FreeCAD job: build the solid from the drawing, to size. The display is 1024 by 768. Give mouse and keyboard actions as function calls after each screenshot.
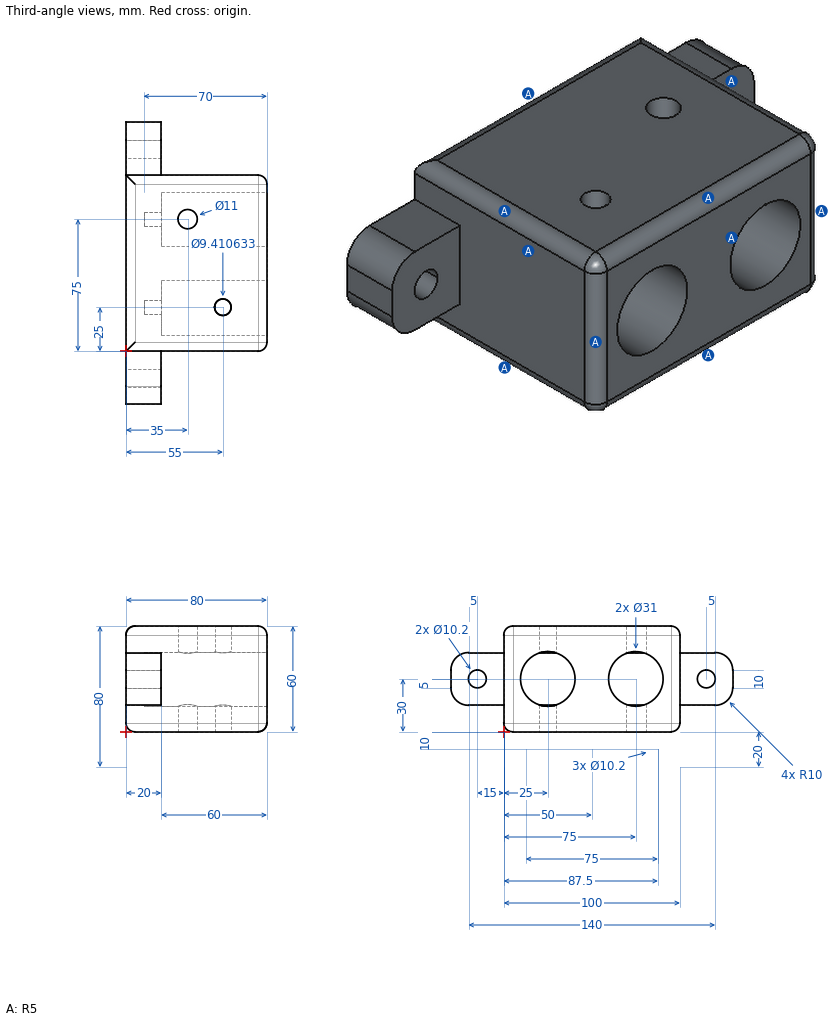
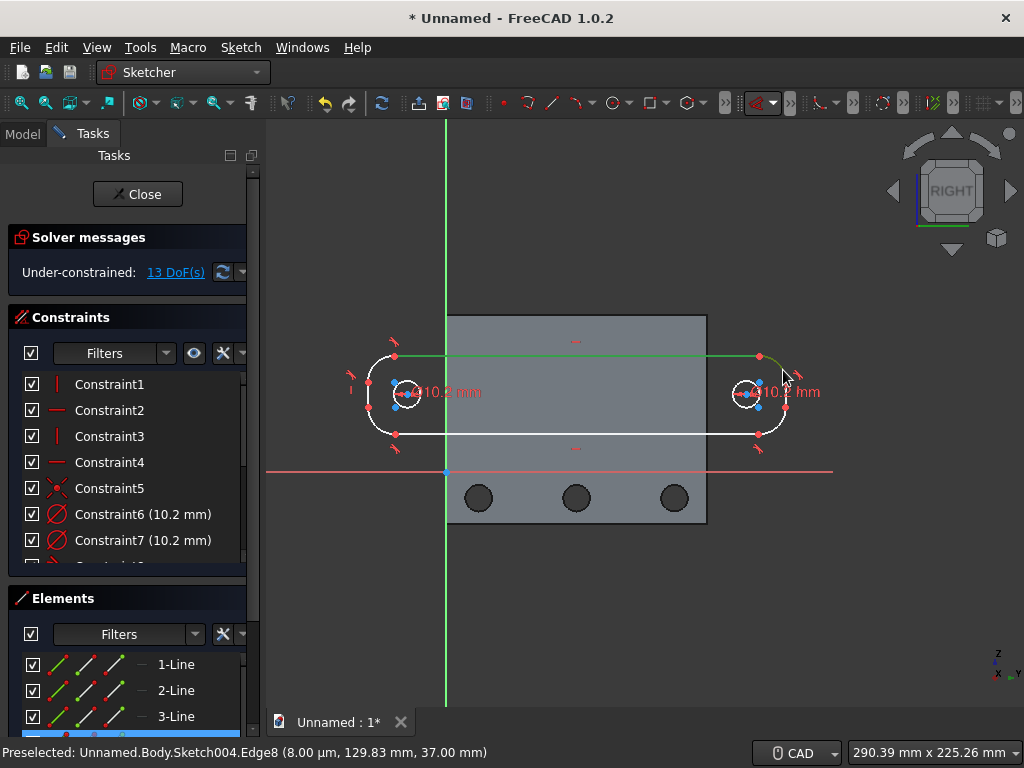
key(t)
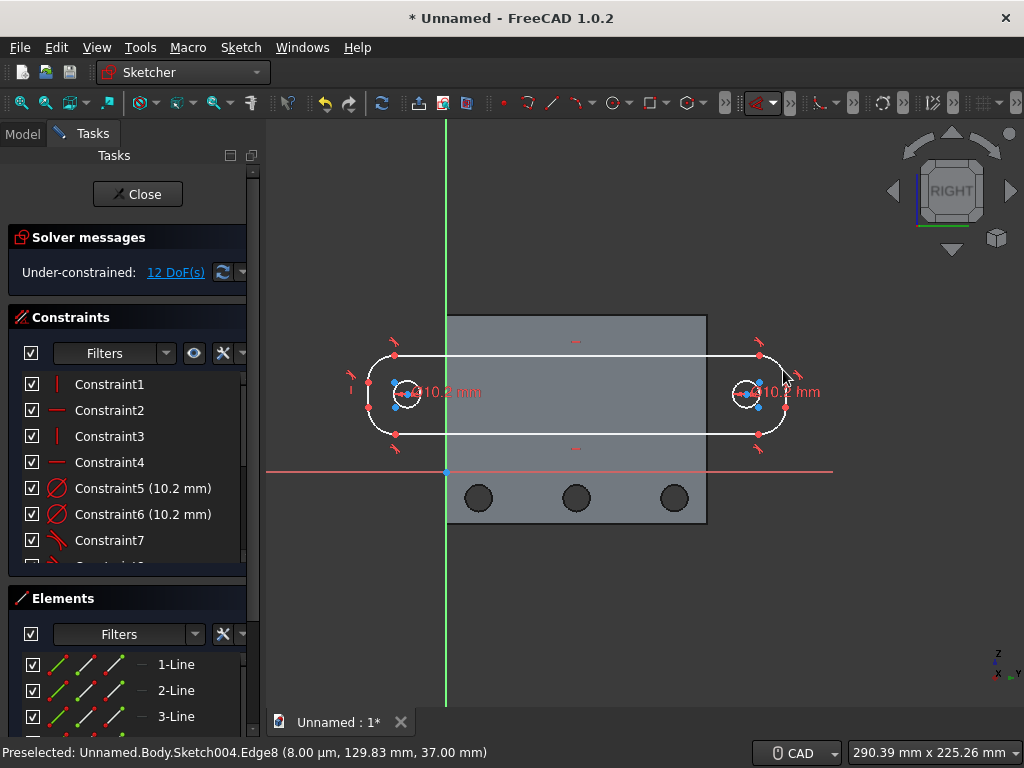
click(771, 431)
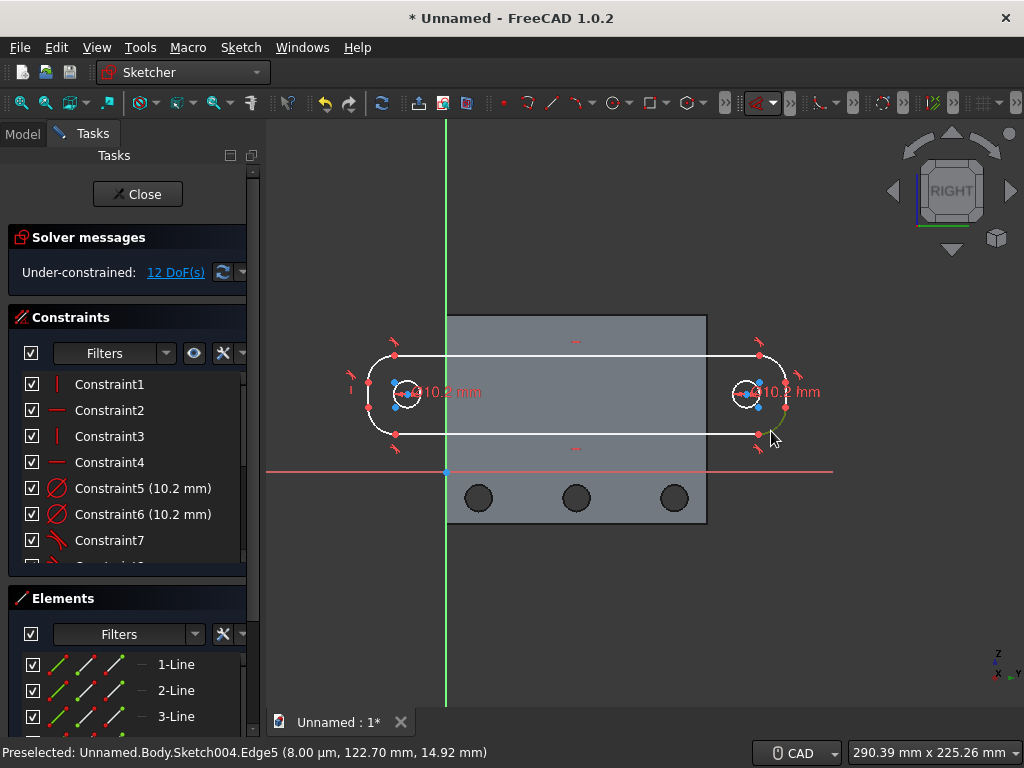
click(371, 419)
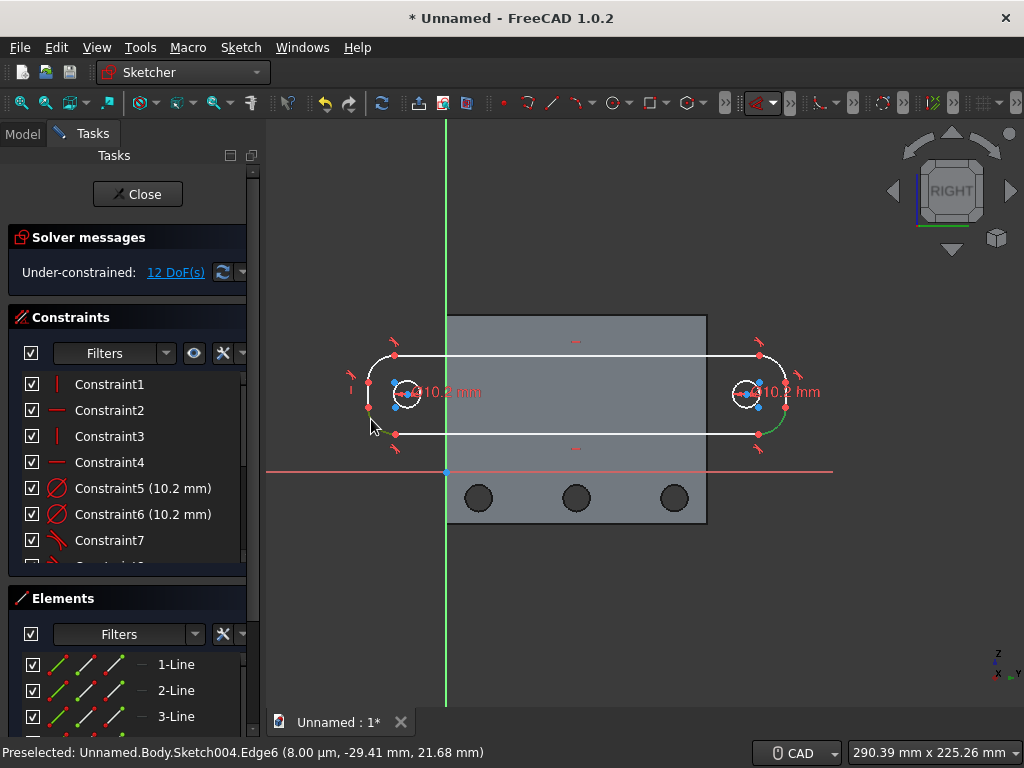
click(382, 359)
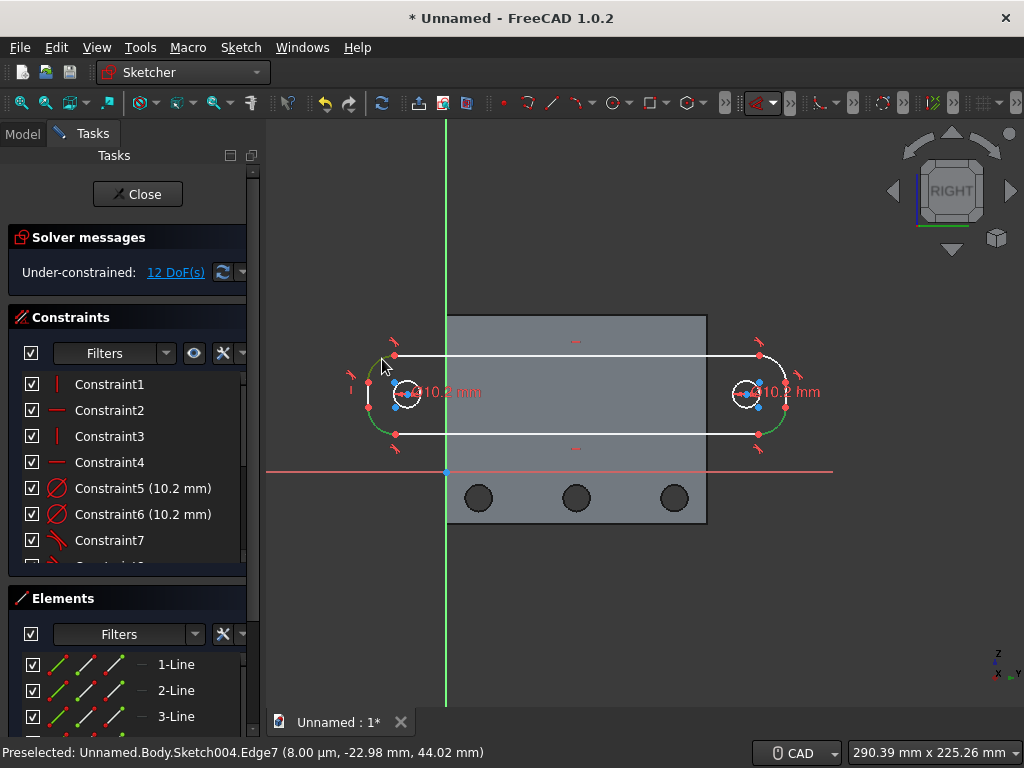
click(783, 370)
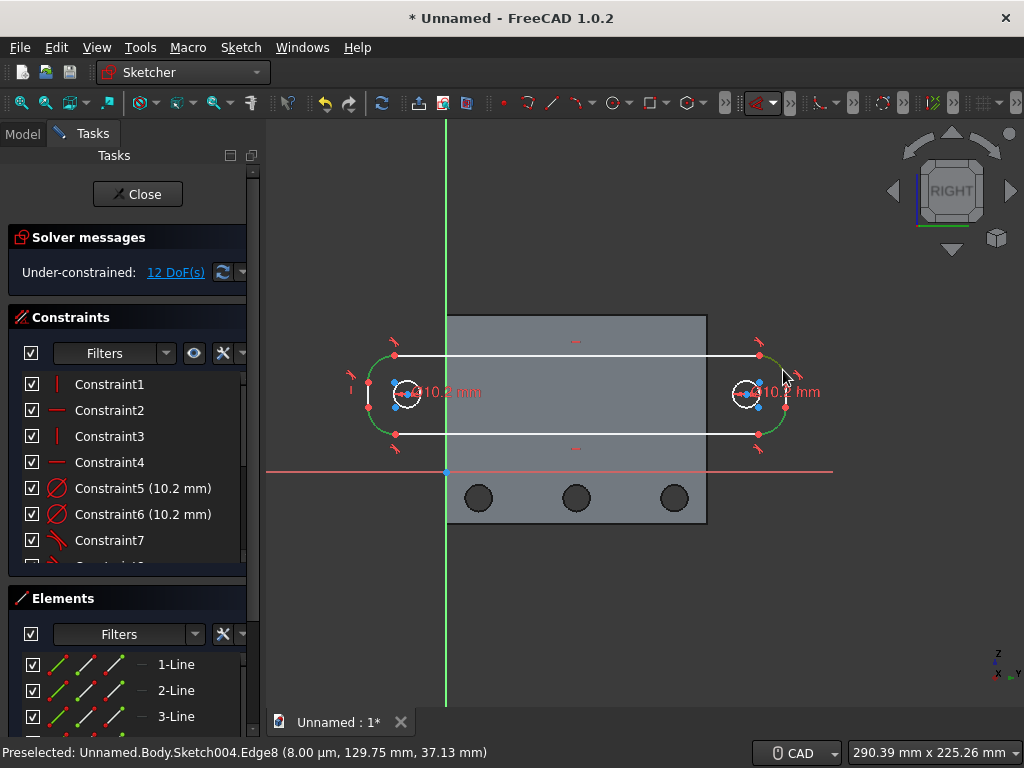
key(e)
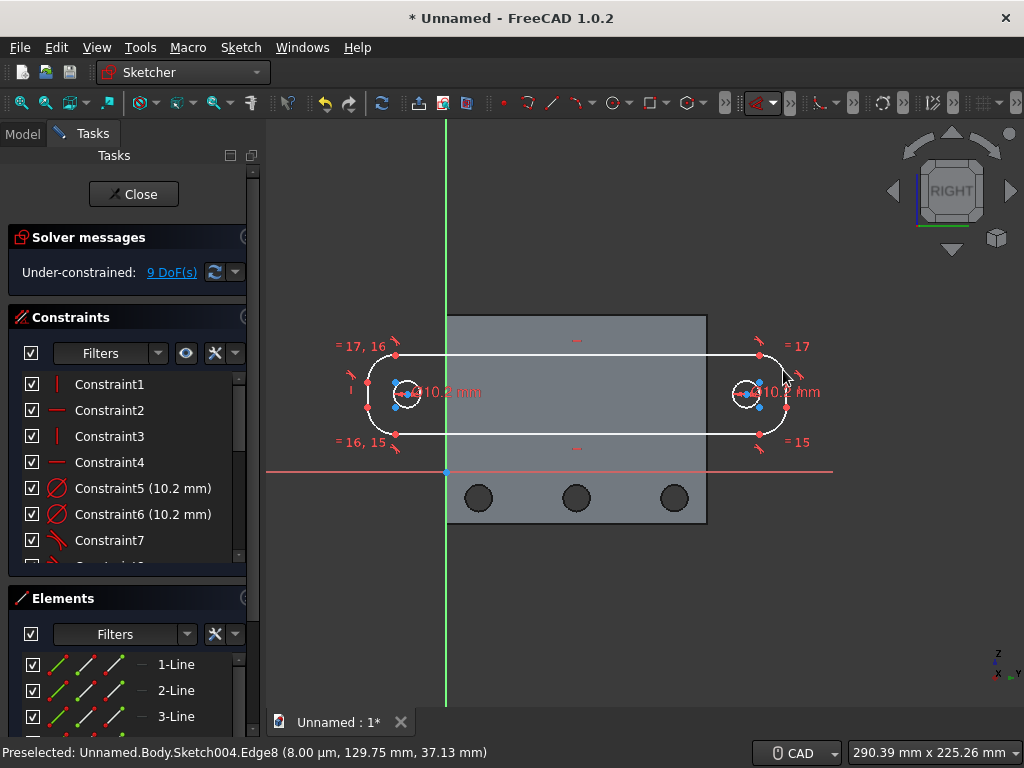
scroll(772, 431, up, 3)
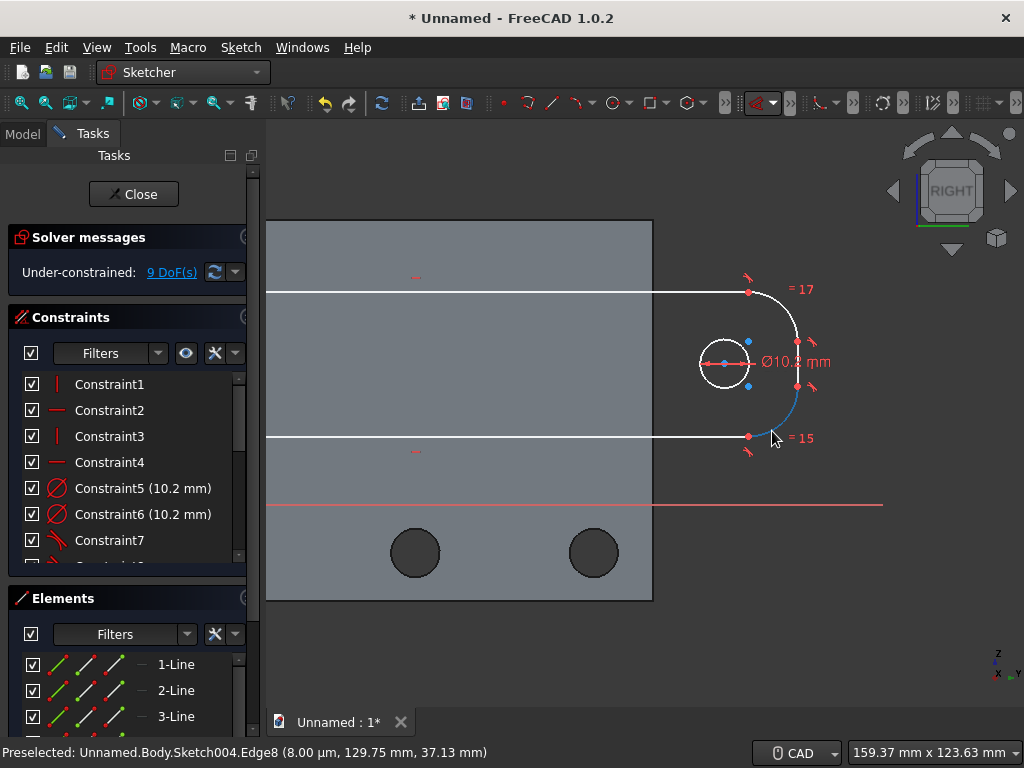
click(771, 431)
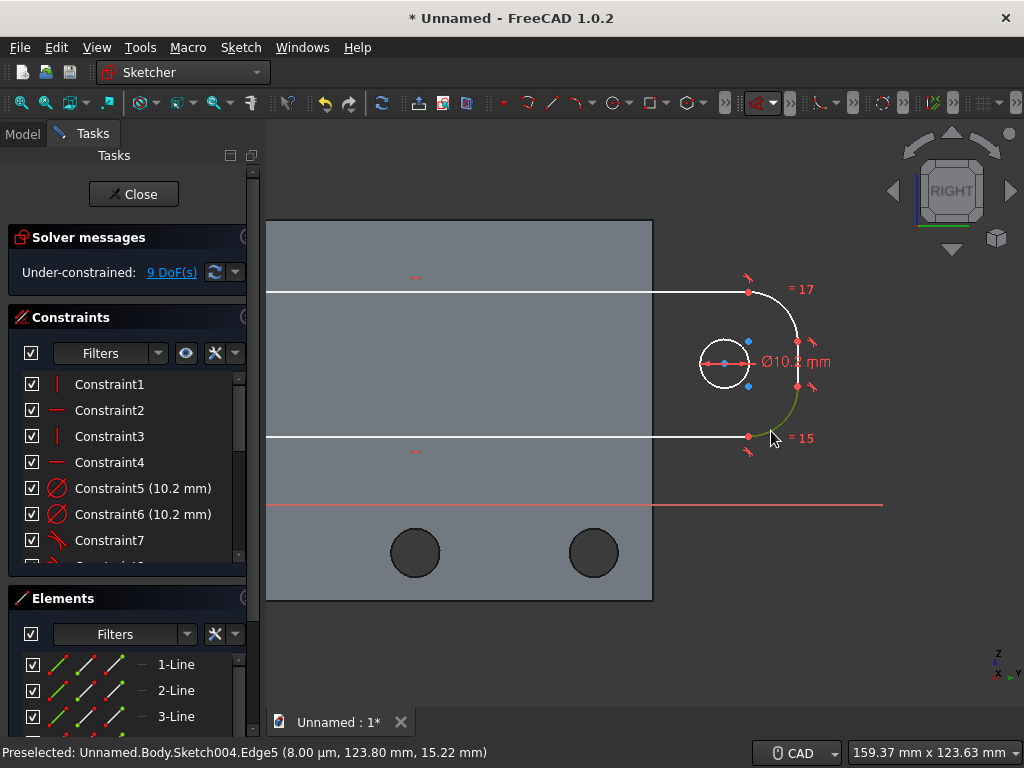
key(k)
key(r)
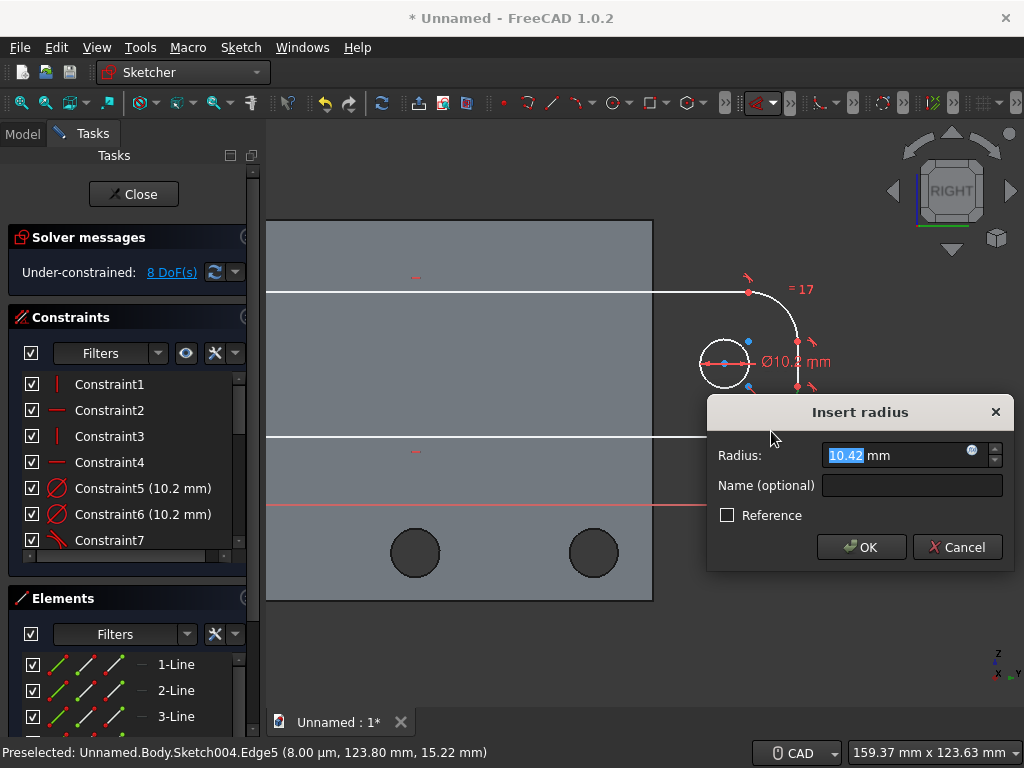
text(10)
key(Return)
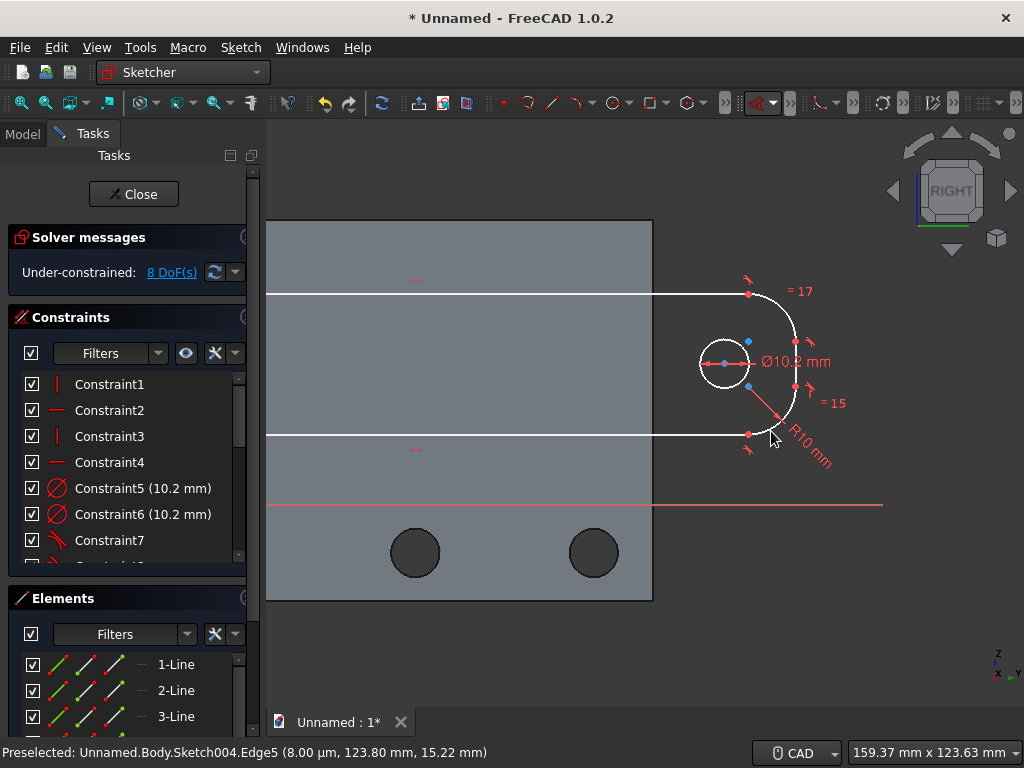
click(796, 355)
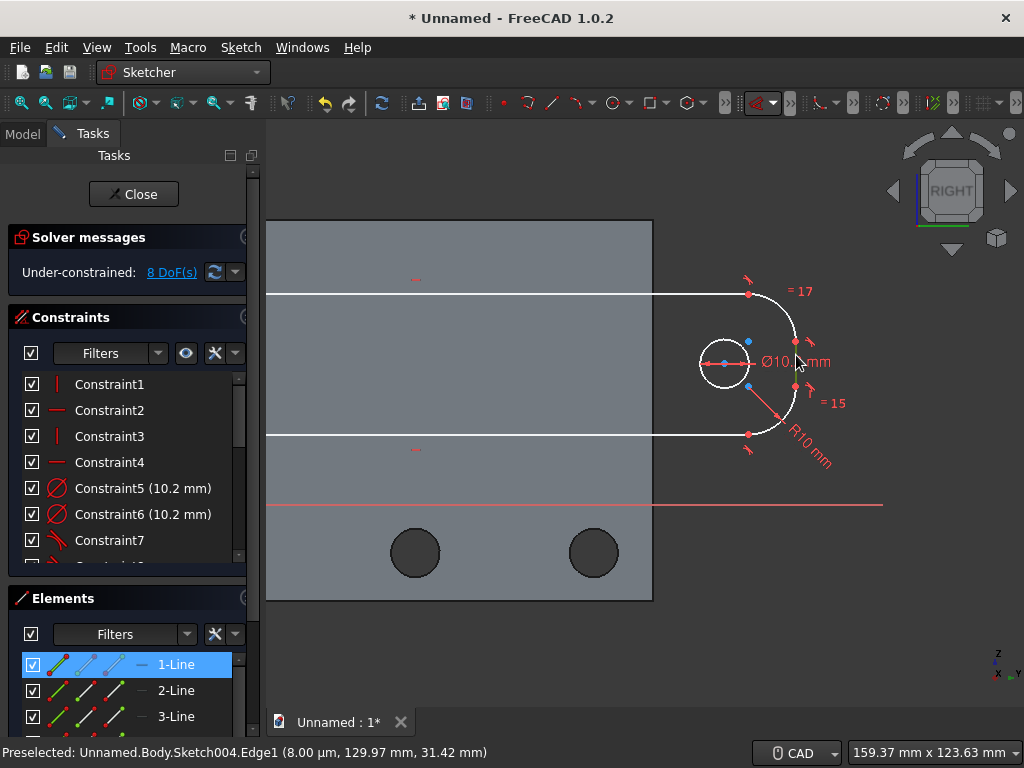
key(i)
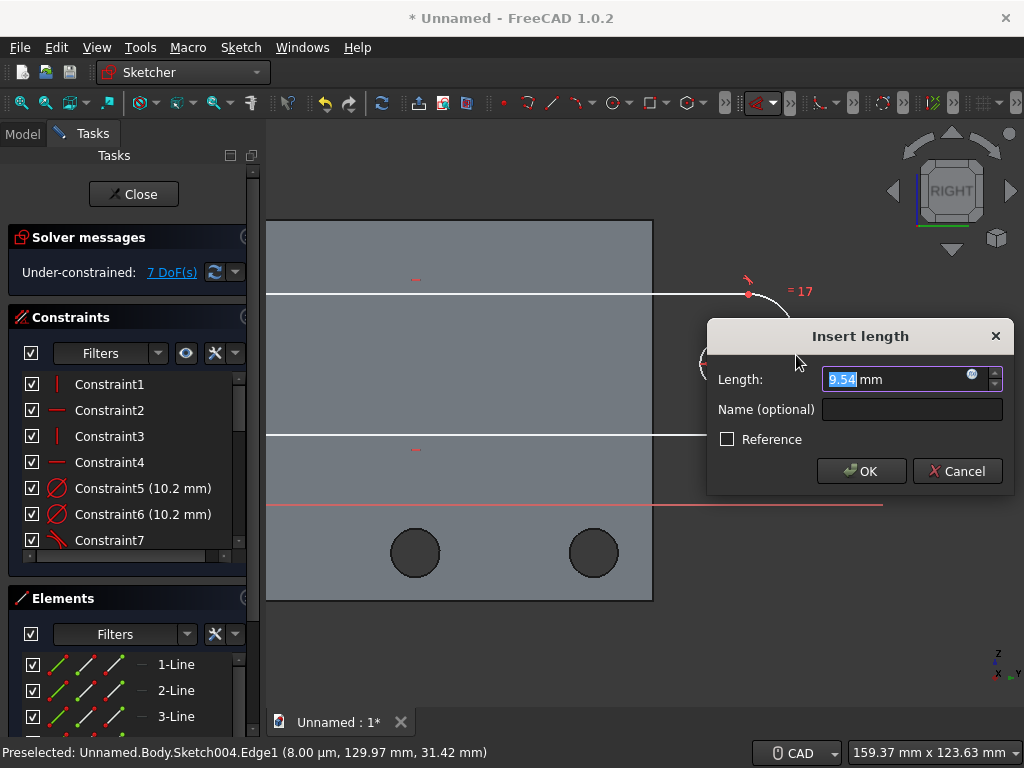
text(10)
key(Return)